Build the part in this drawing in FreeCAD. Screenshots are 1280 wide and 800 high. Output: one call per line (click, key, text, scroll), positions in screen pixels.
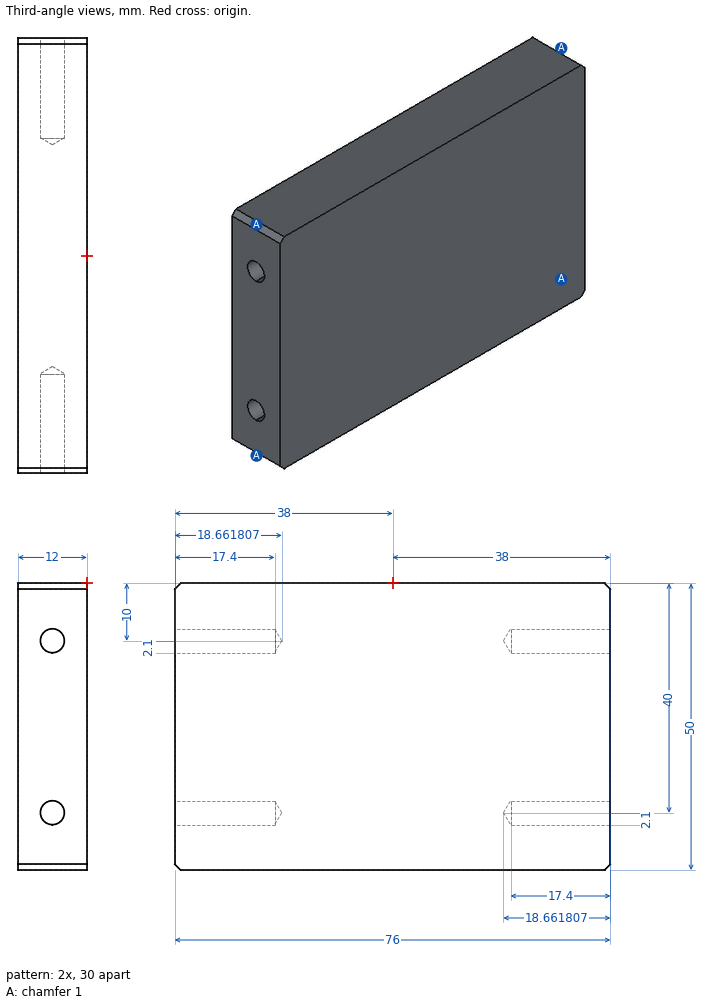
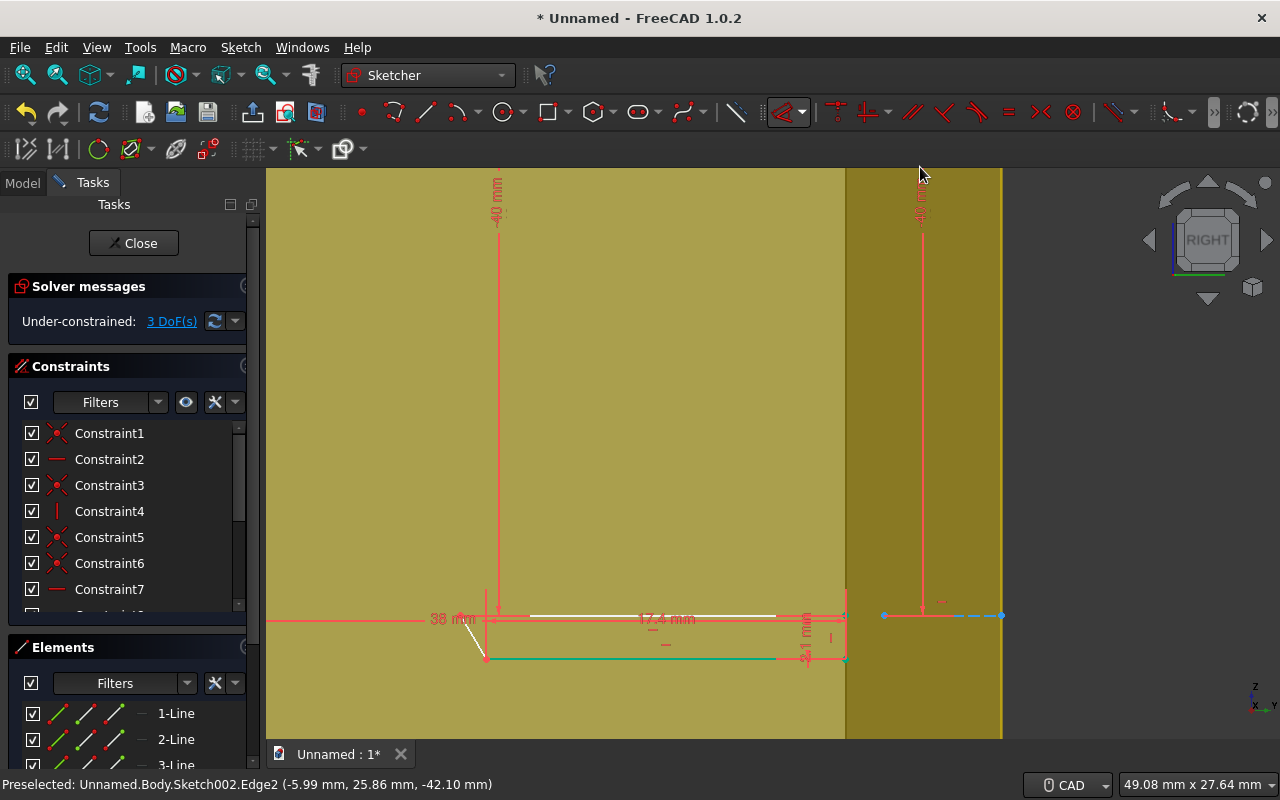
click(730, 616)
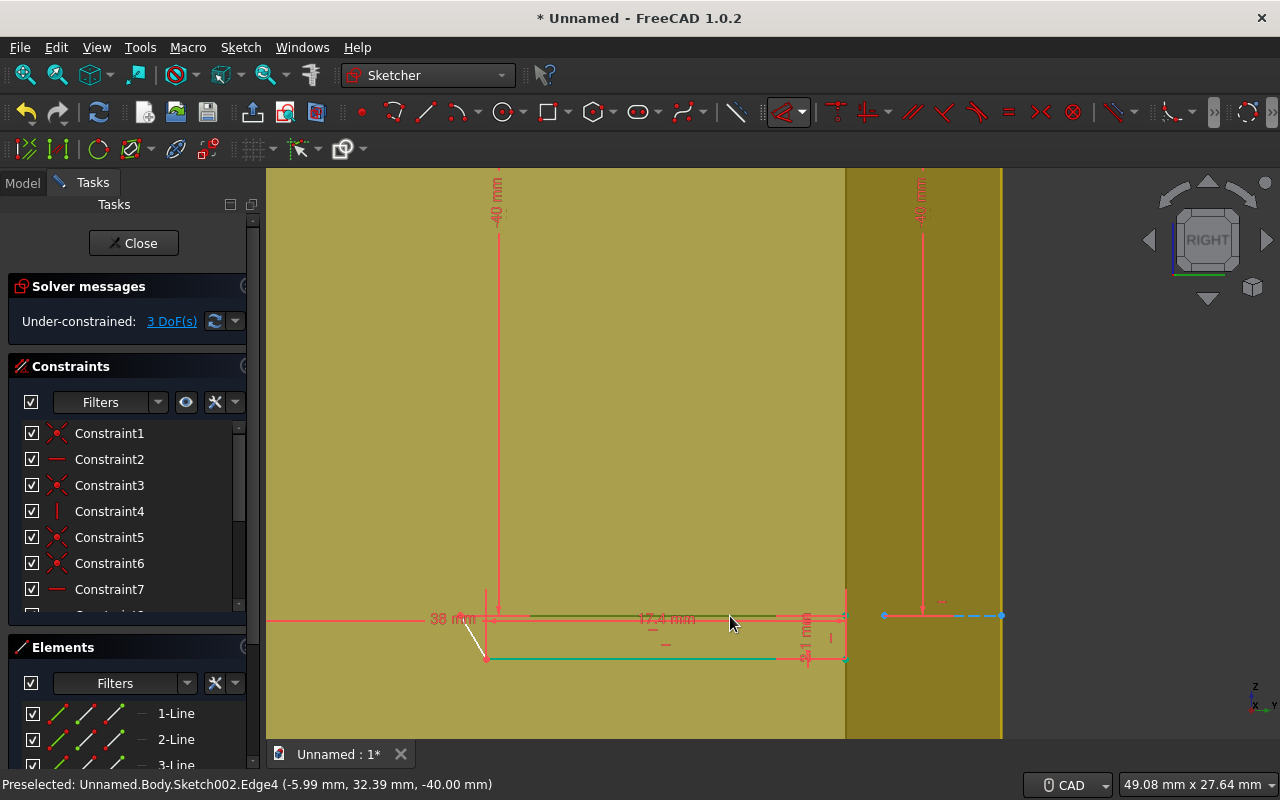
click(804, 112)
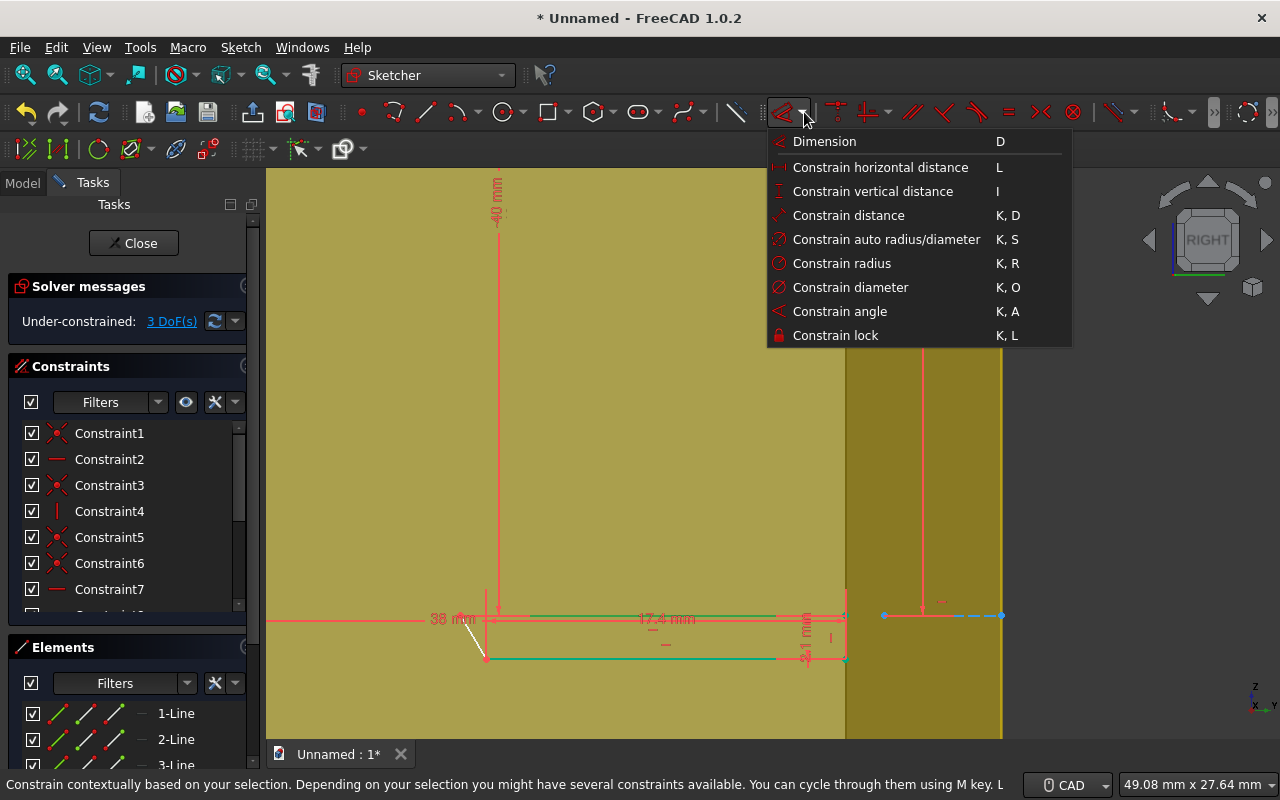
click(920, 167)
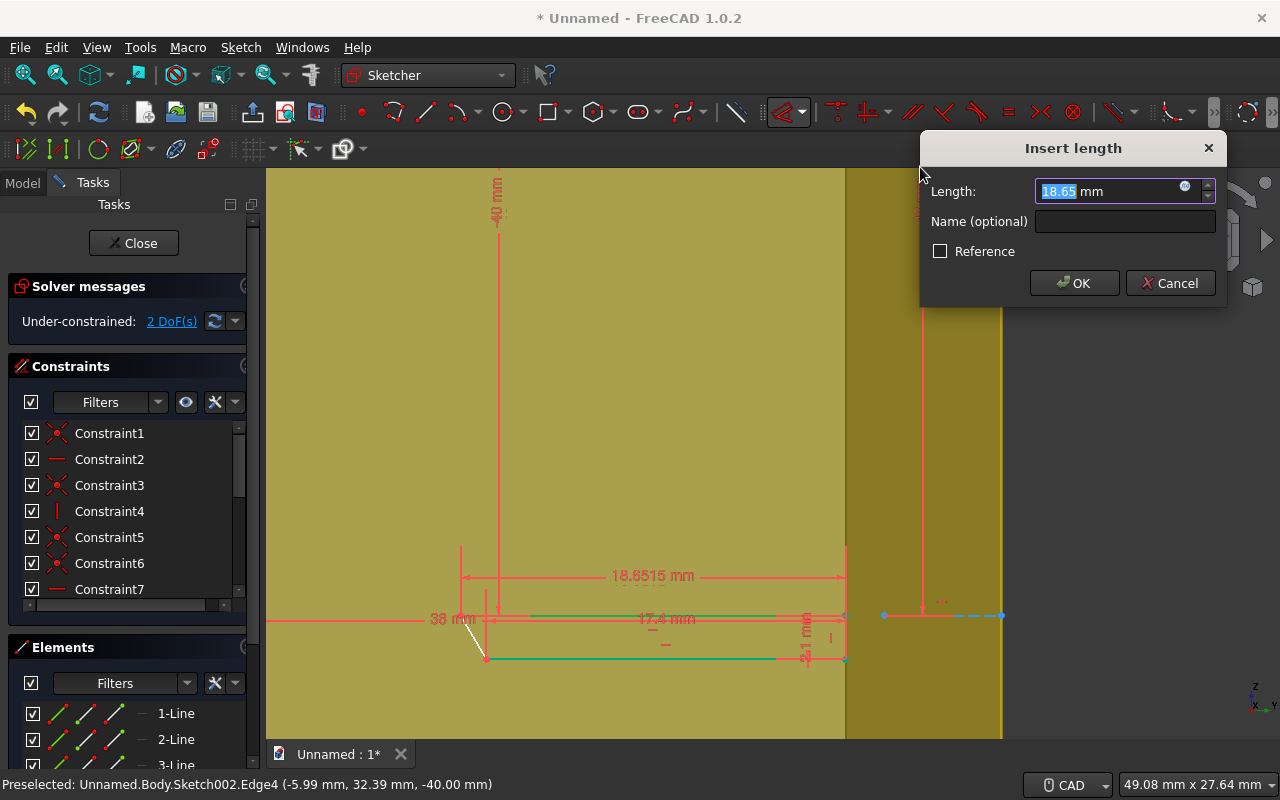
text(18.661807)
key(Return)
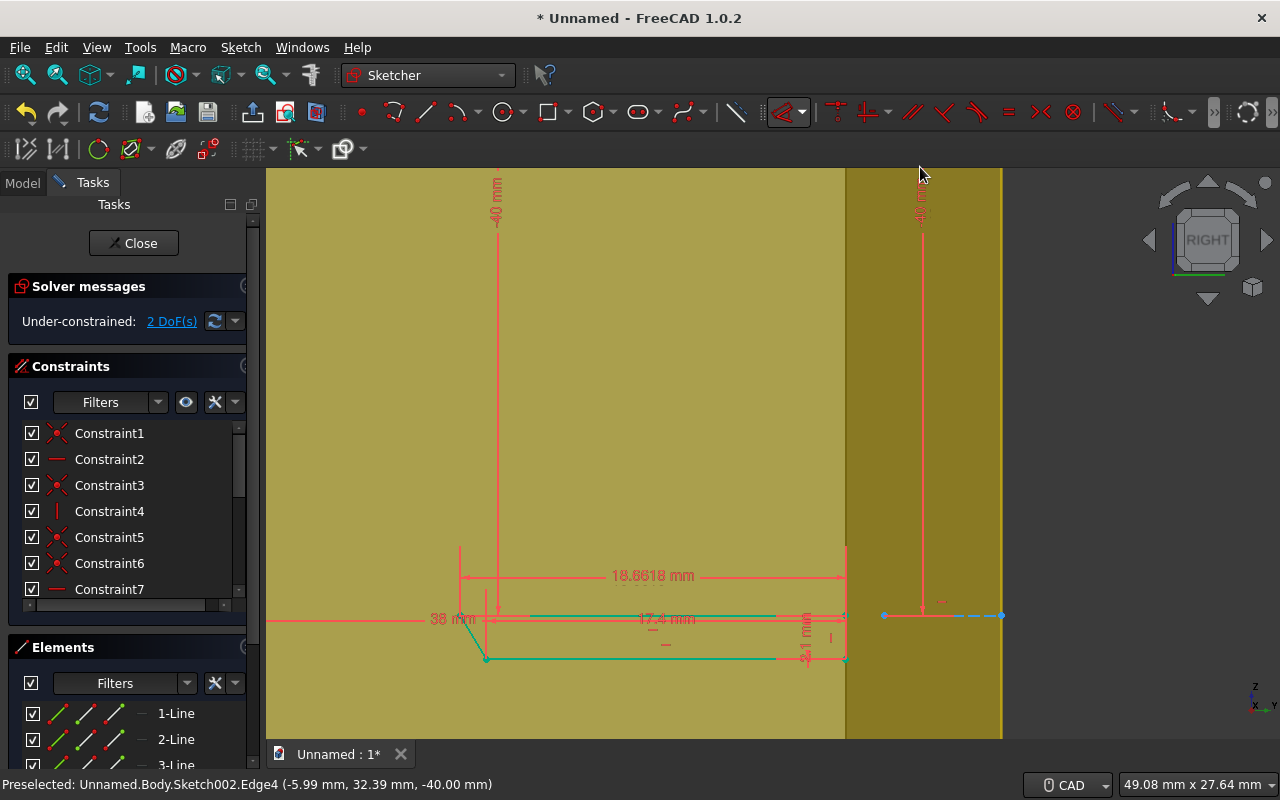
click(134, 243)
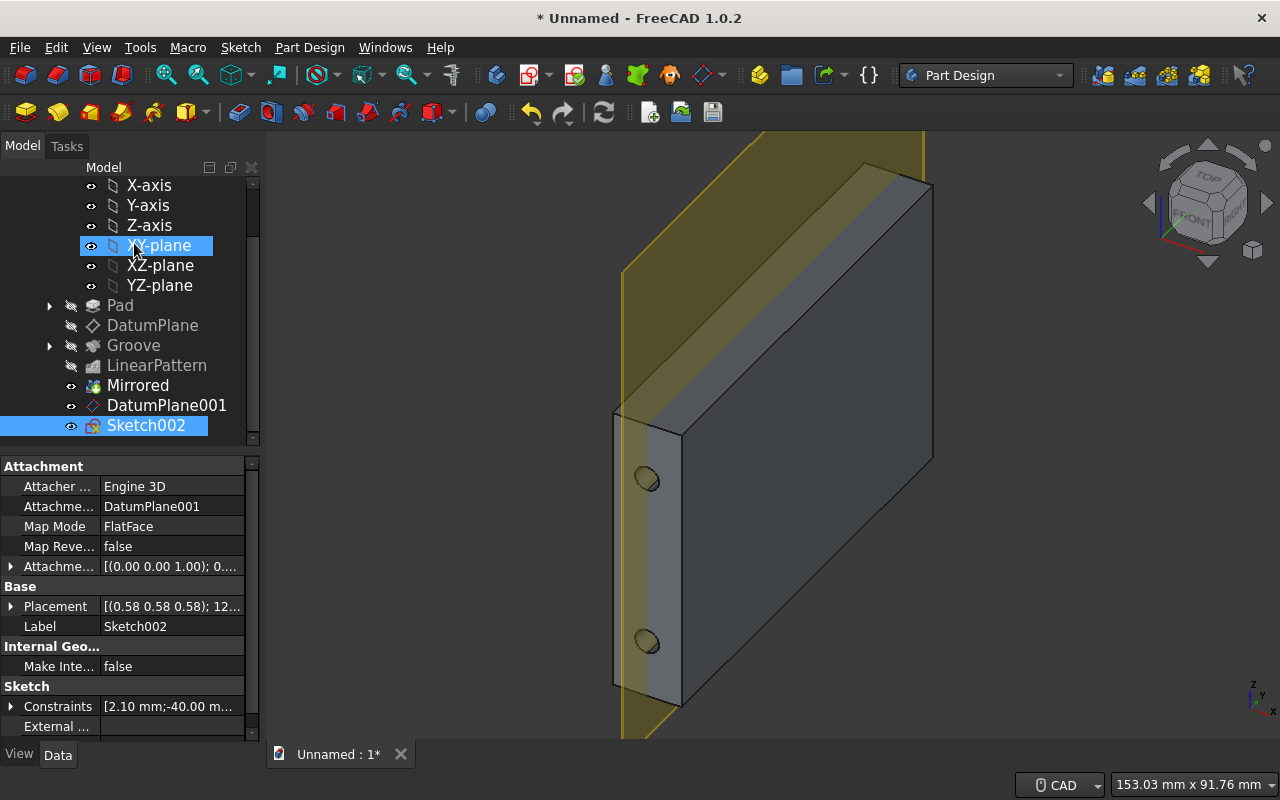
click(304, 112)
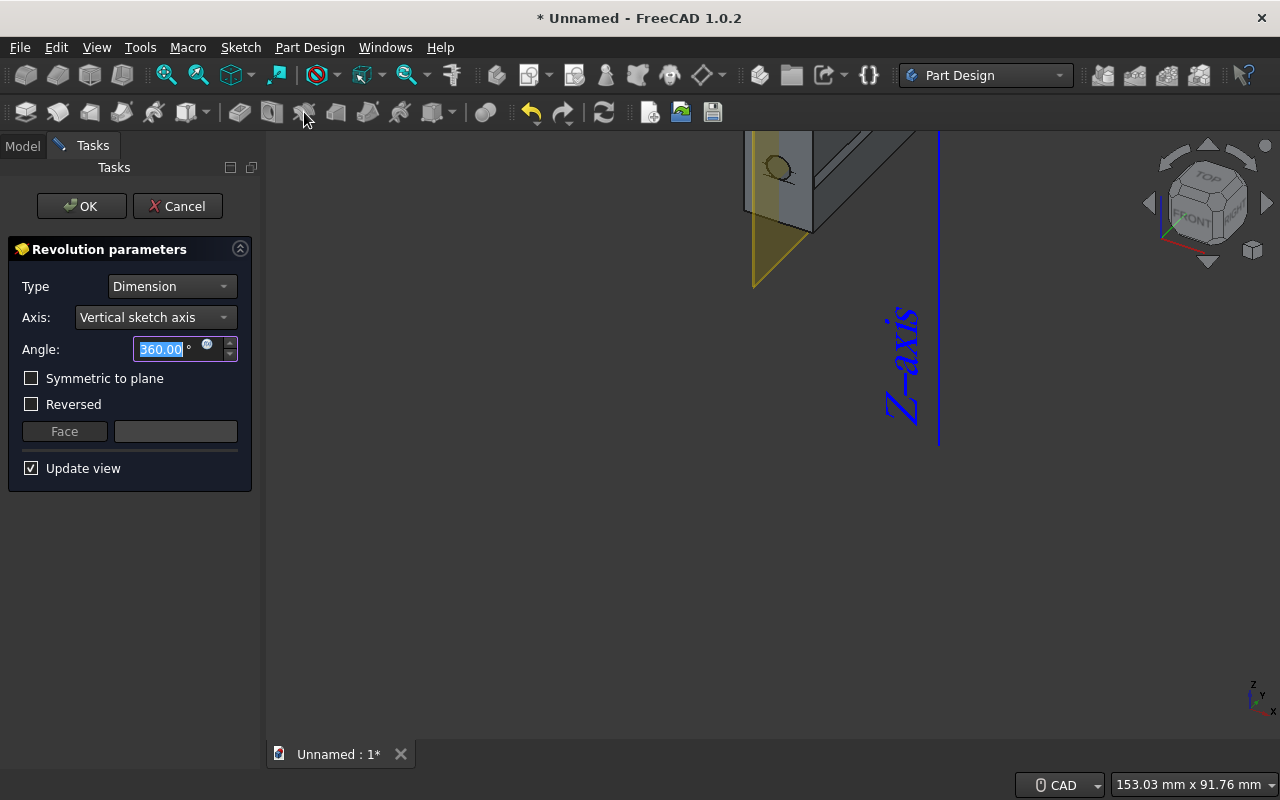
click(156, 318)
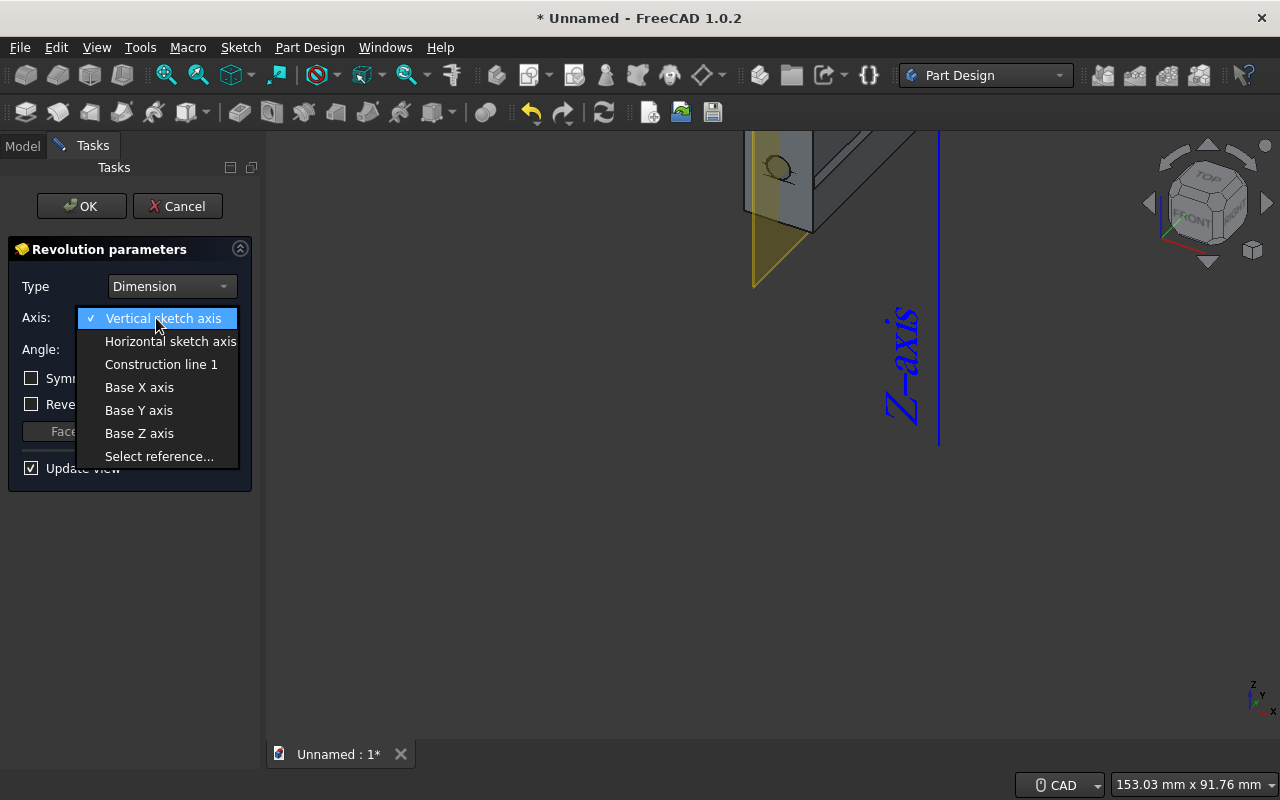
click(156, 364)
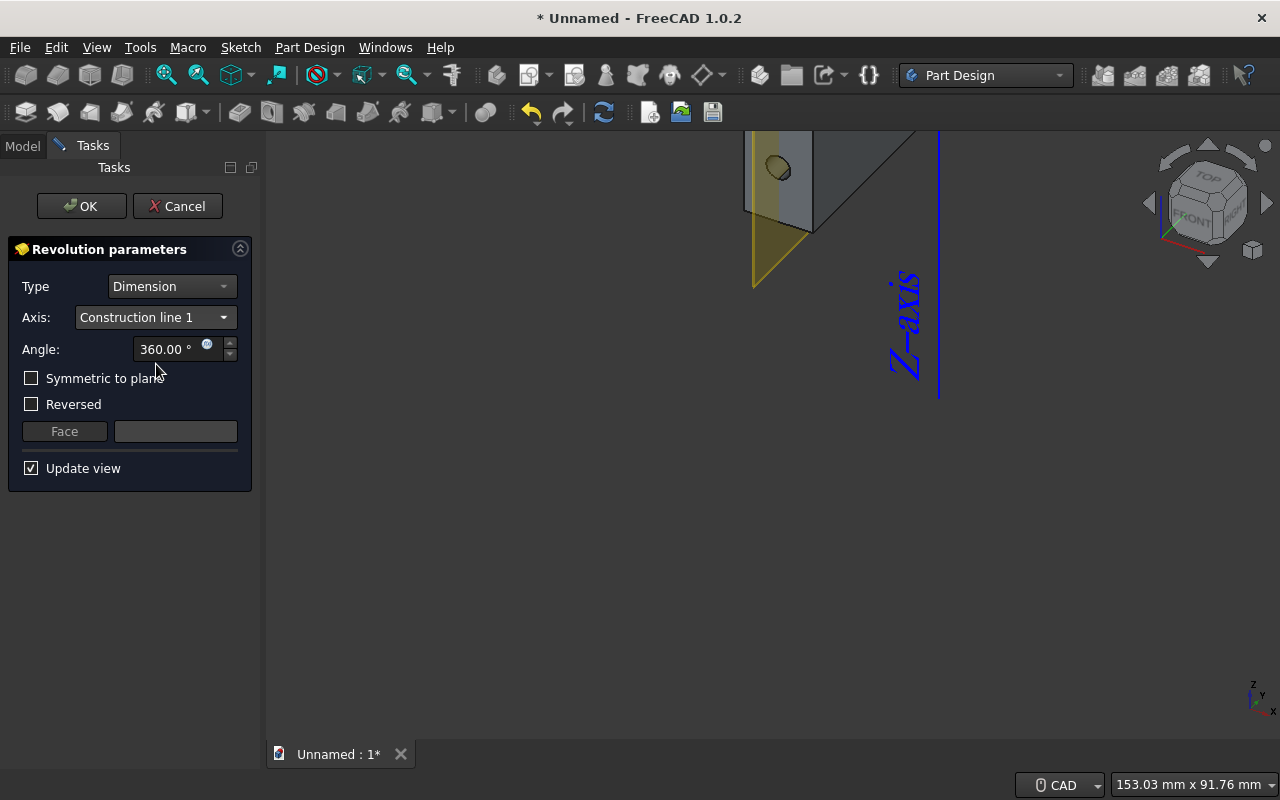
click(82, 206)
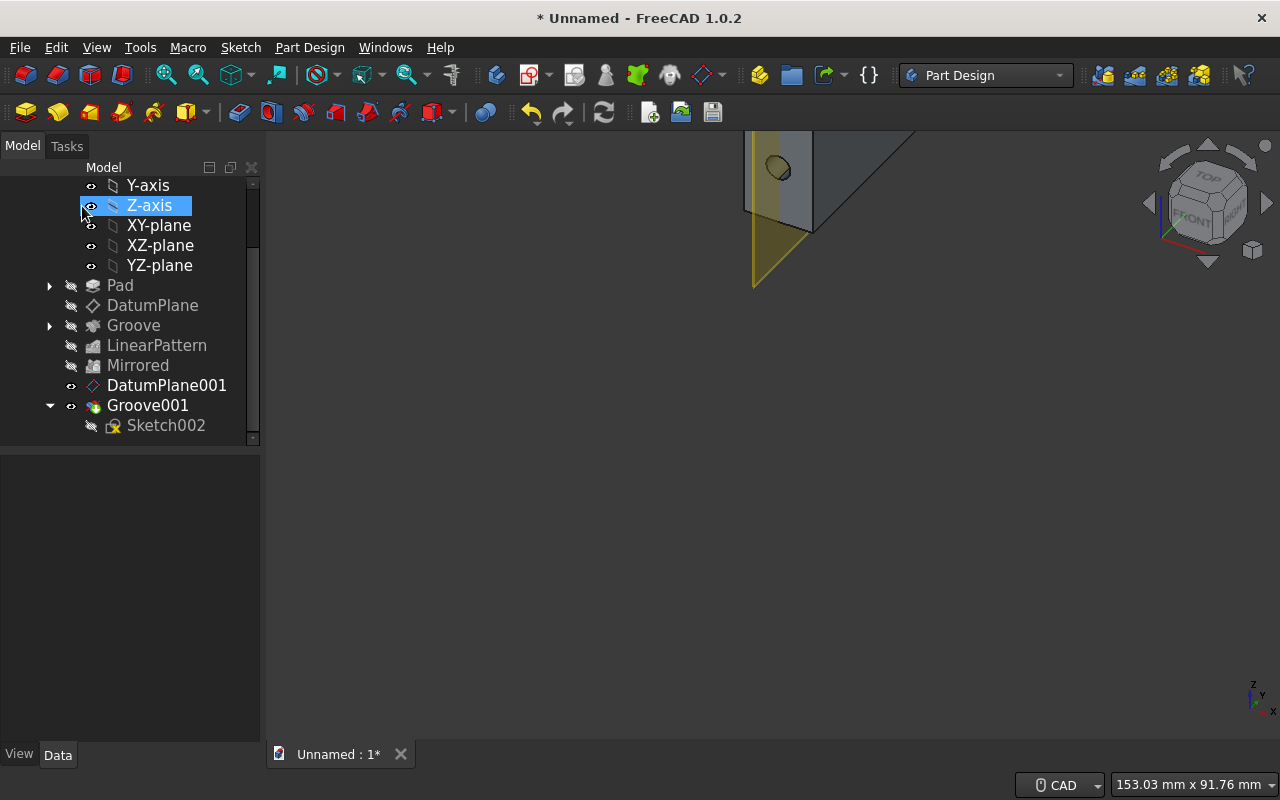
click(116, 386)
key(space)